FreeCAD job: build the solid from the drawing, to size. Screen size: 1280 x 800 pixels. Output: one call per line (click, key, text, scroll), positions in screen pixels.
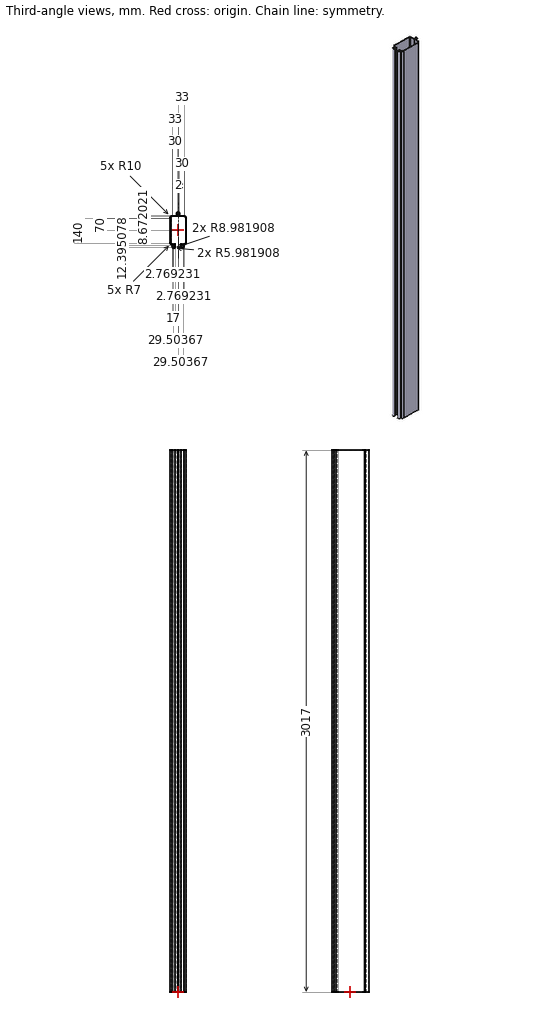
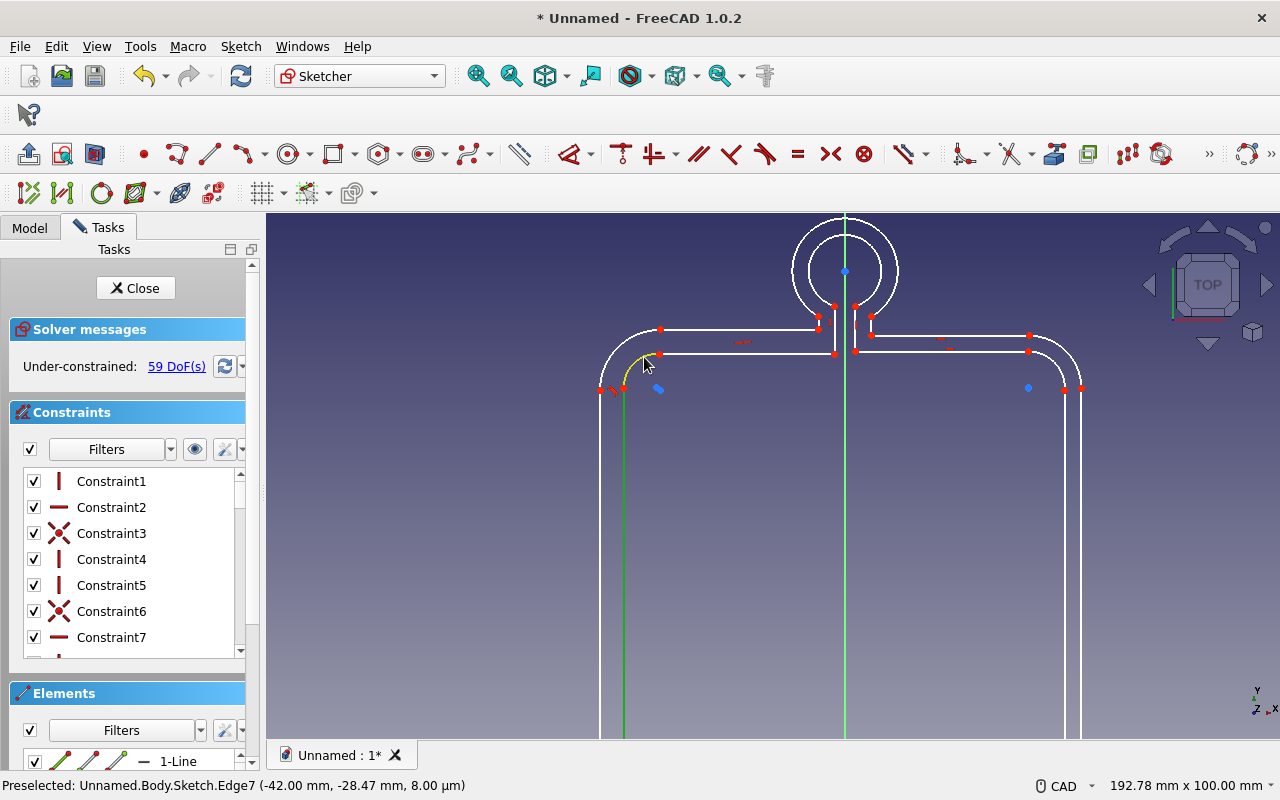
click(643, 357)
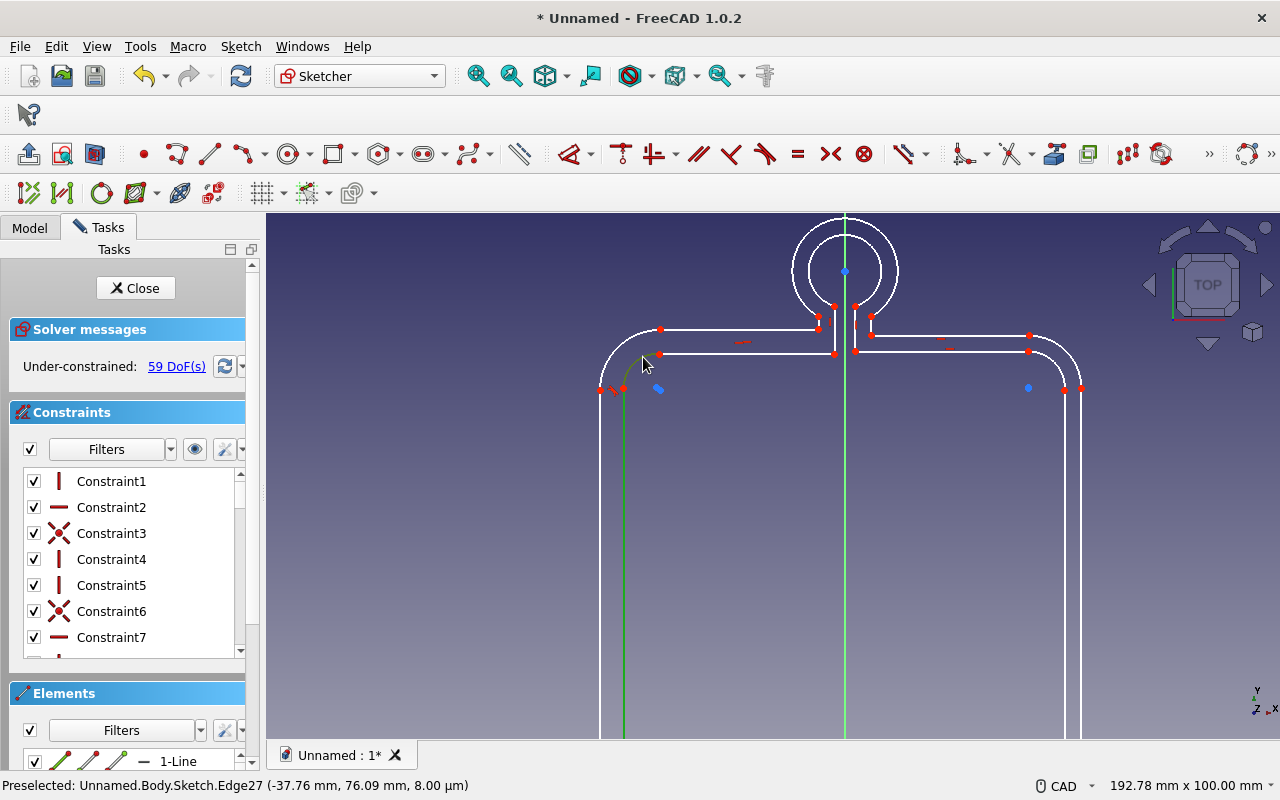
click(765, 154)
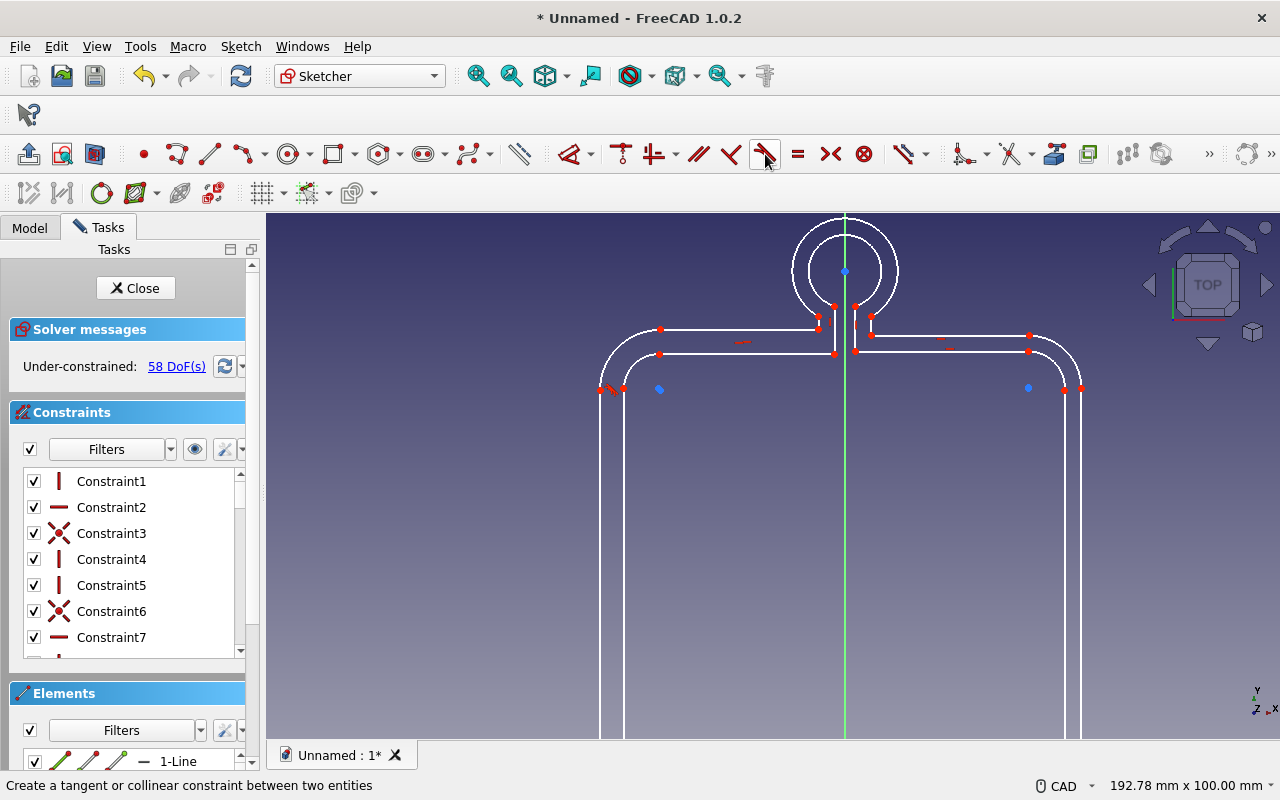
click(712, 354)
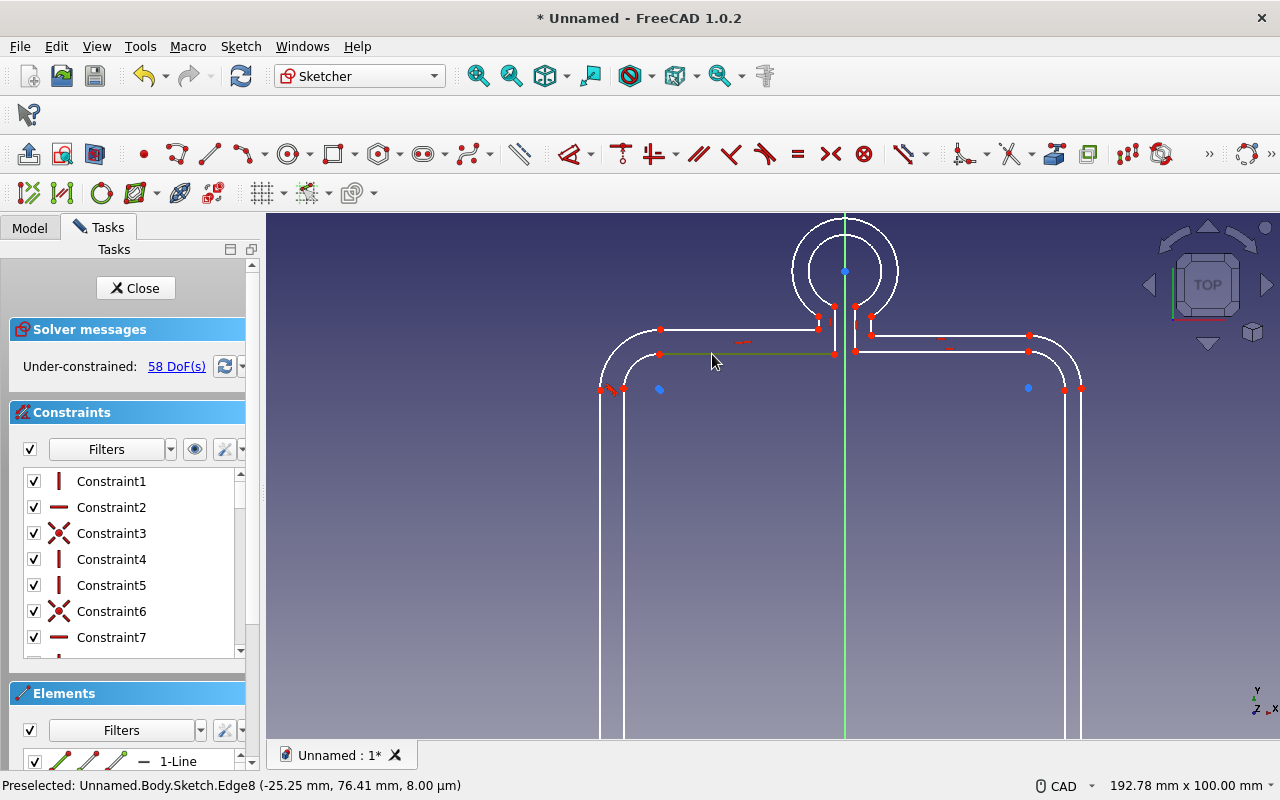
click(643, 358)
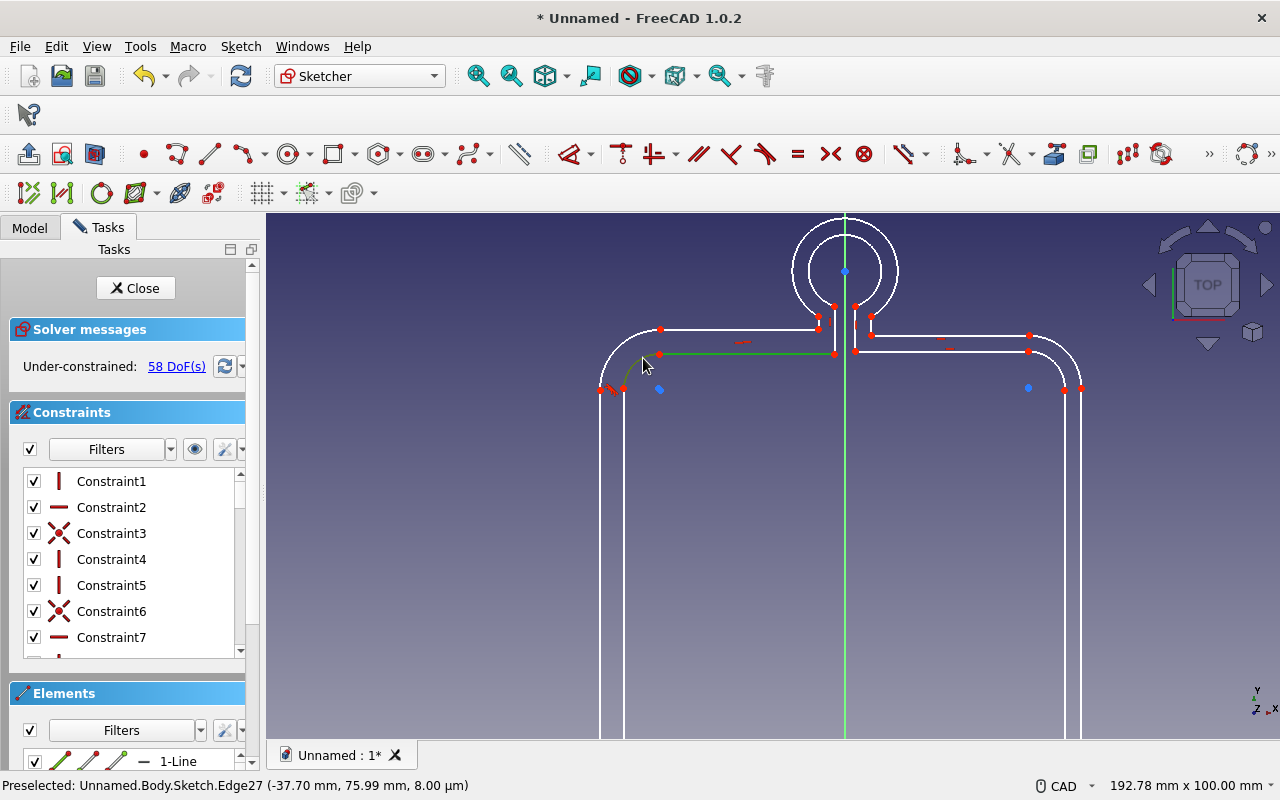
click(765, 154)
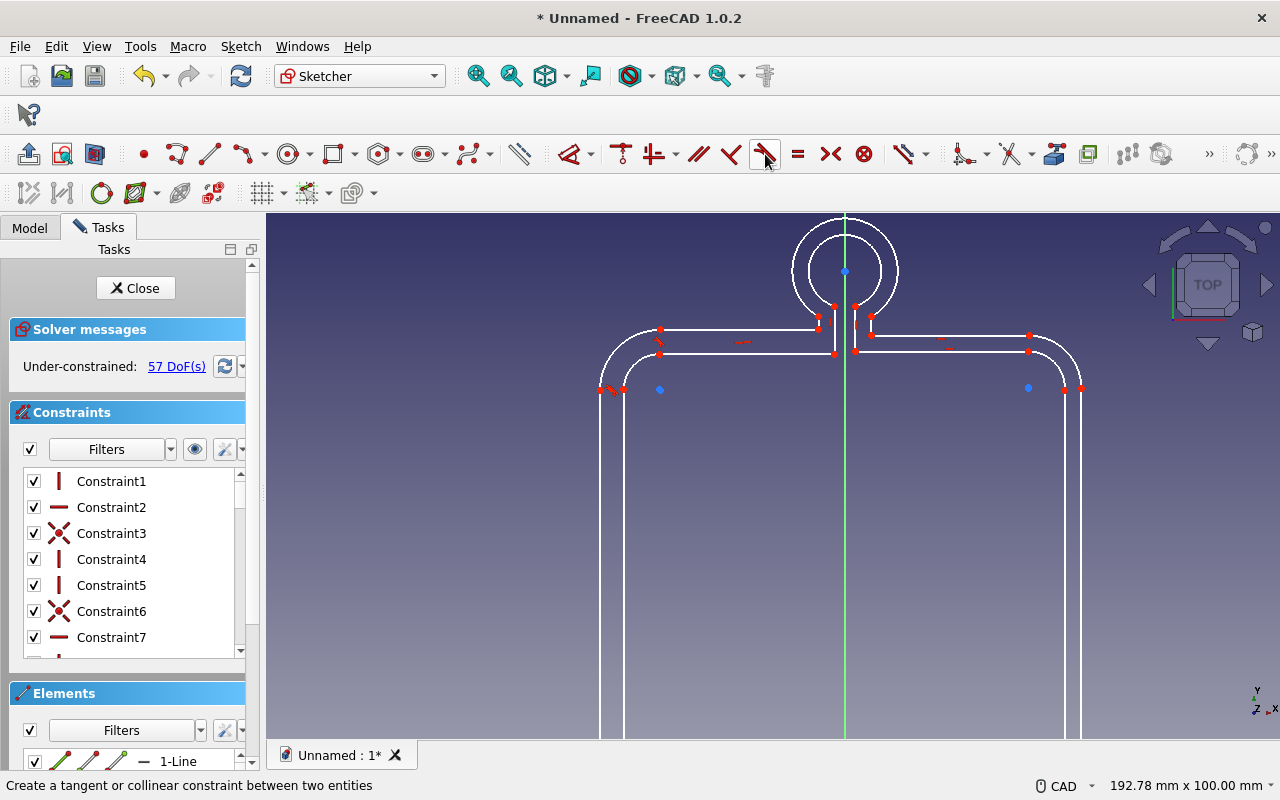
click(907, 352)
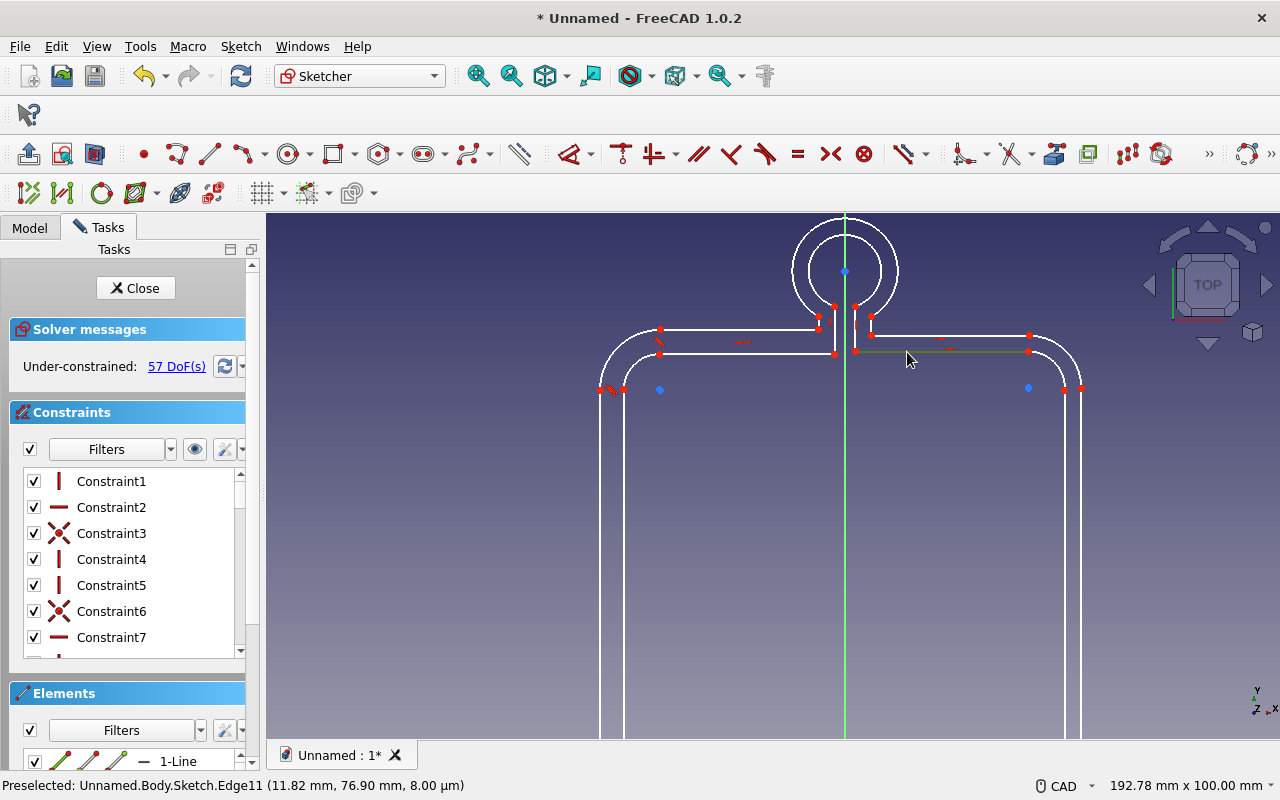
click(1062, 373)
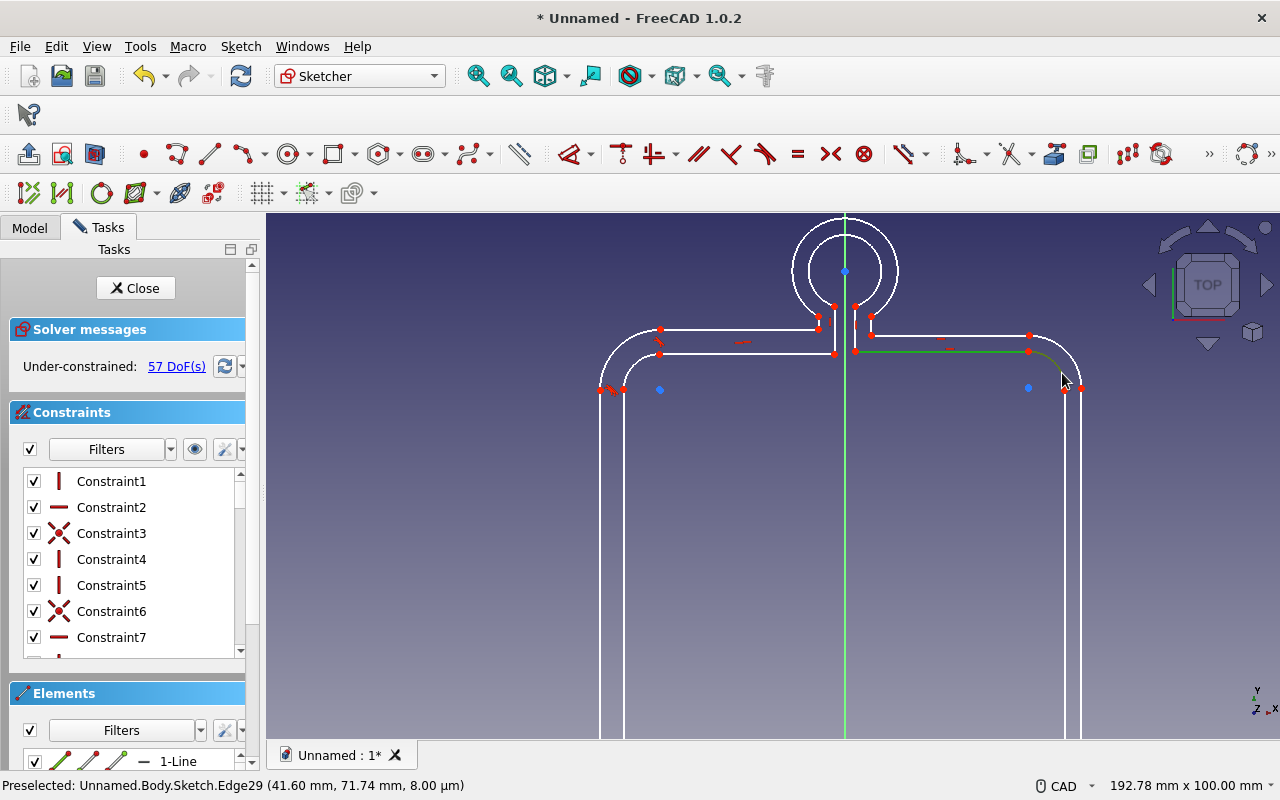
click(765, 154)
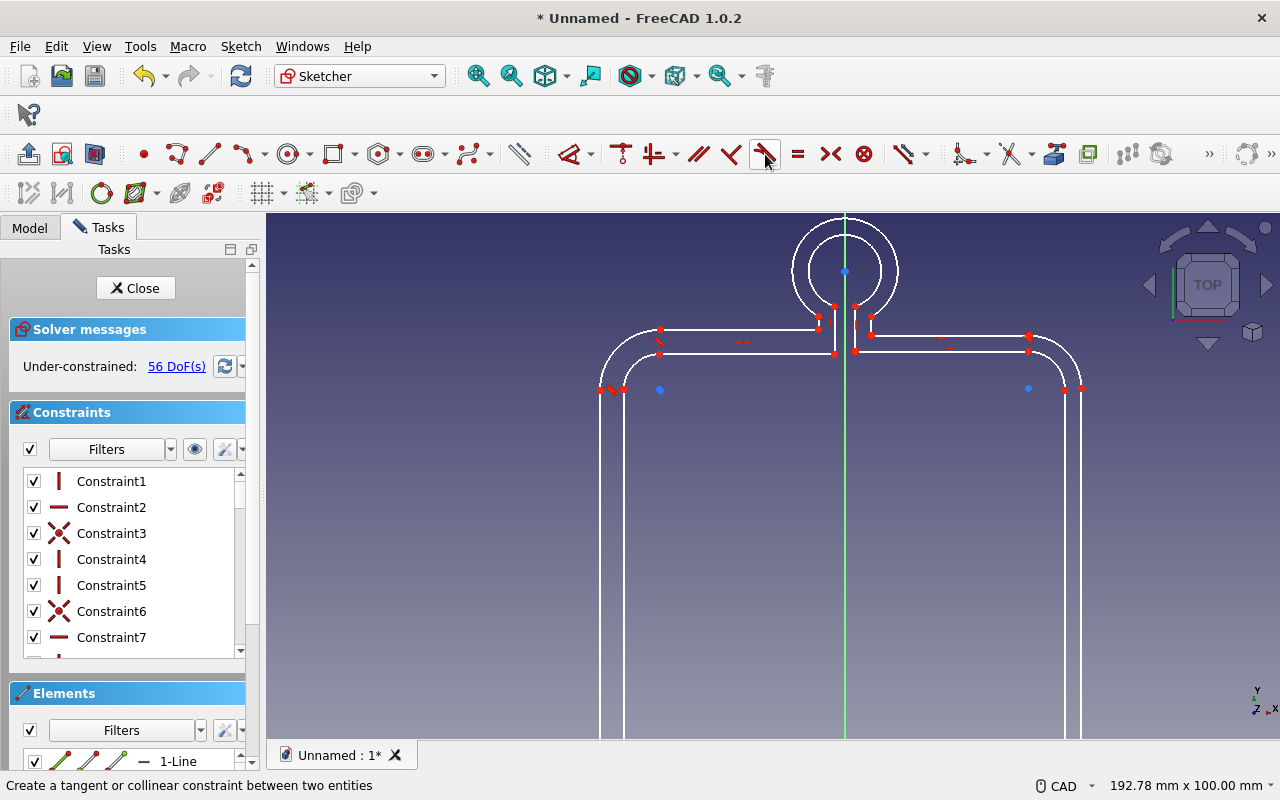
click(1065, 612)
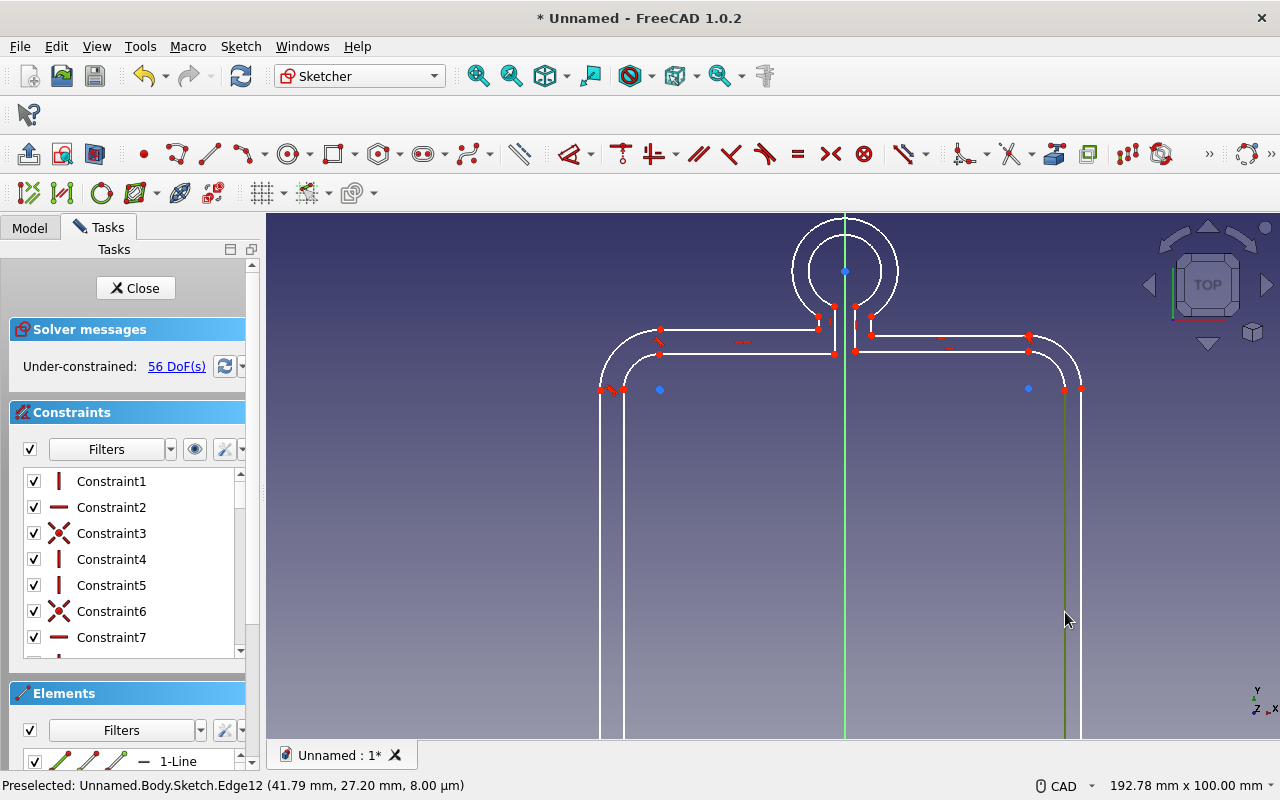
click(1061, 373)